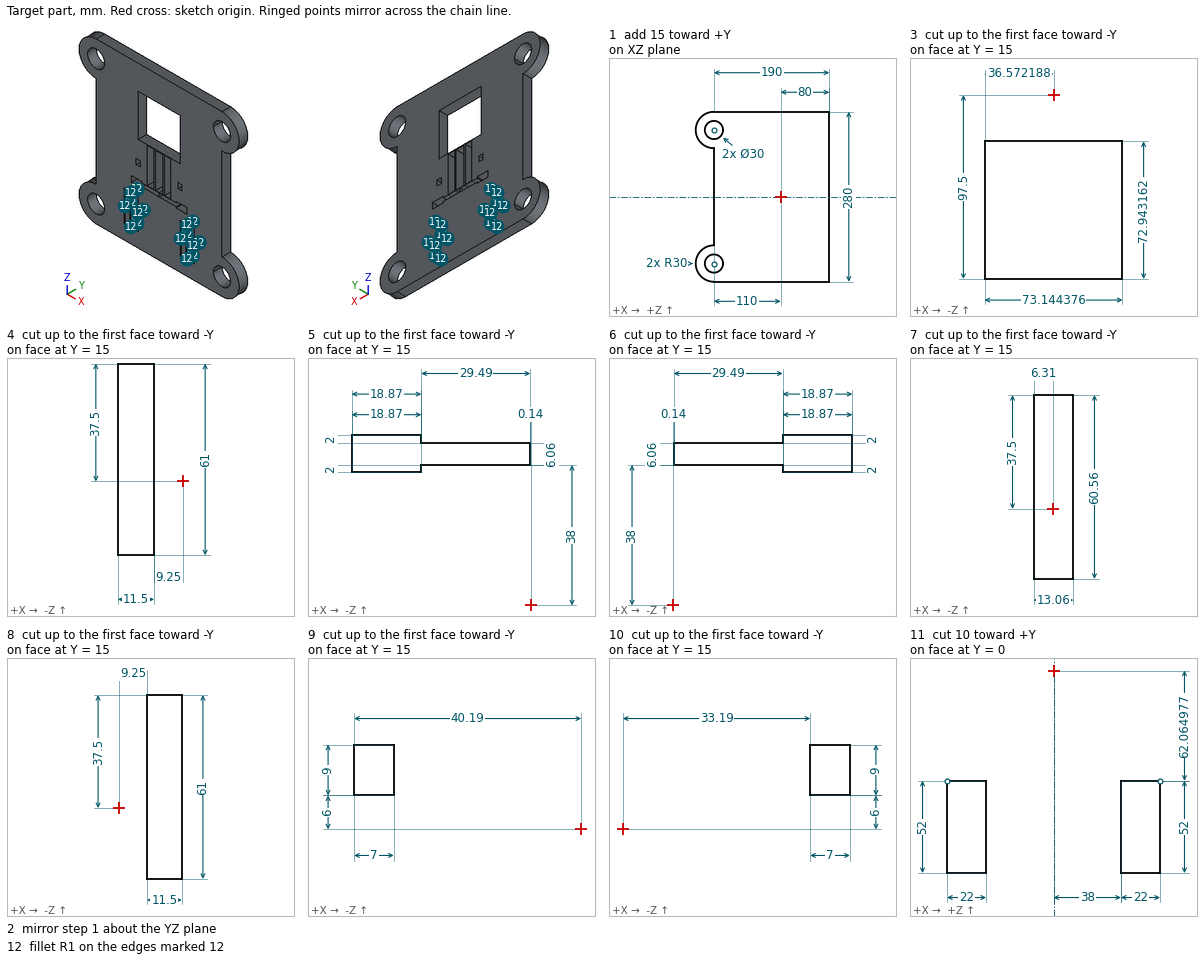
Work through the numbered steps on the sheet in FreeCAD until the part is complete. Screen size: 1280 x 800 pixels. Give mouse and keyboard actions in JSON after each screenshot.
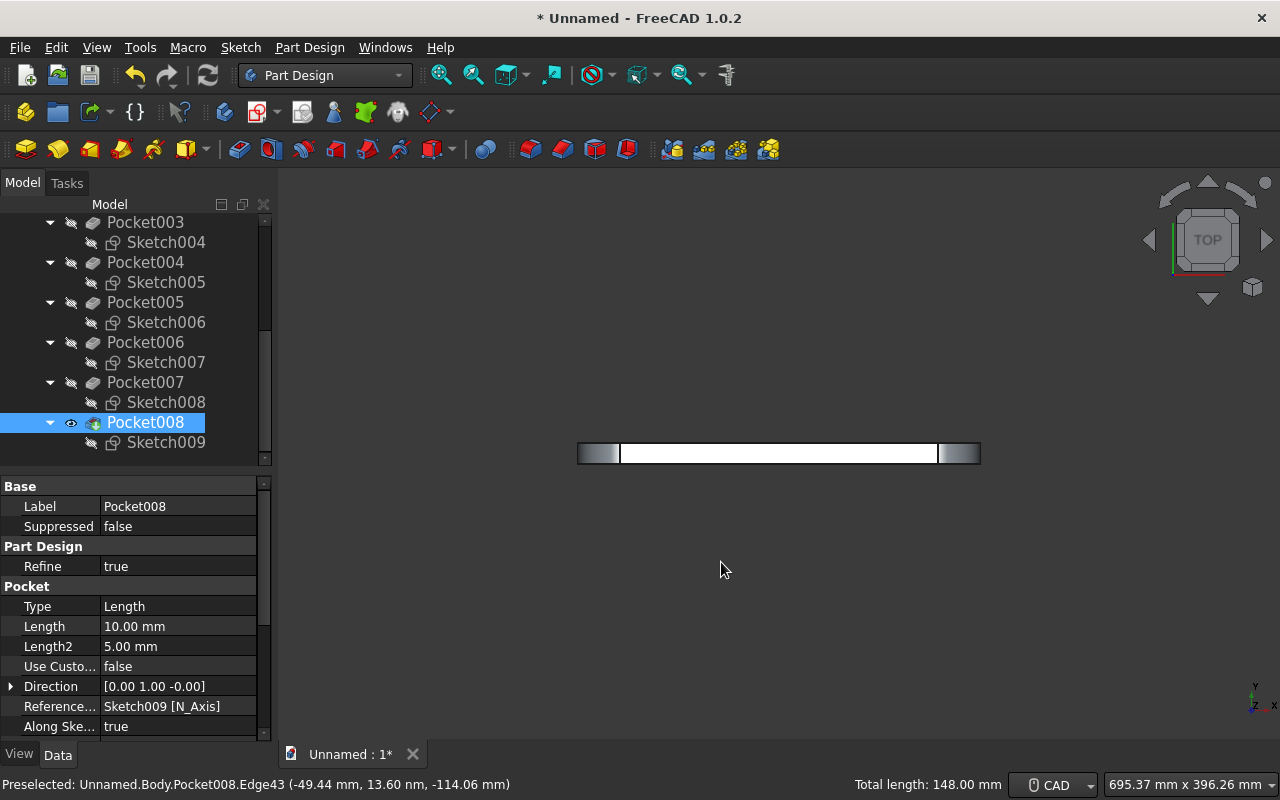
{"action": "left_click", "coordinate": [442, 76]}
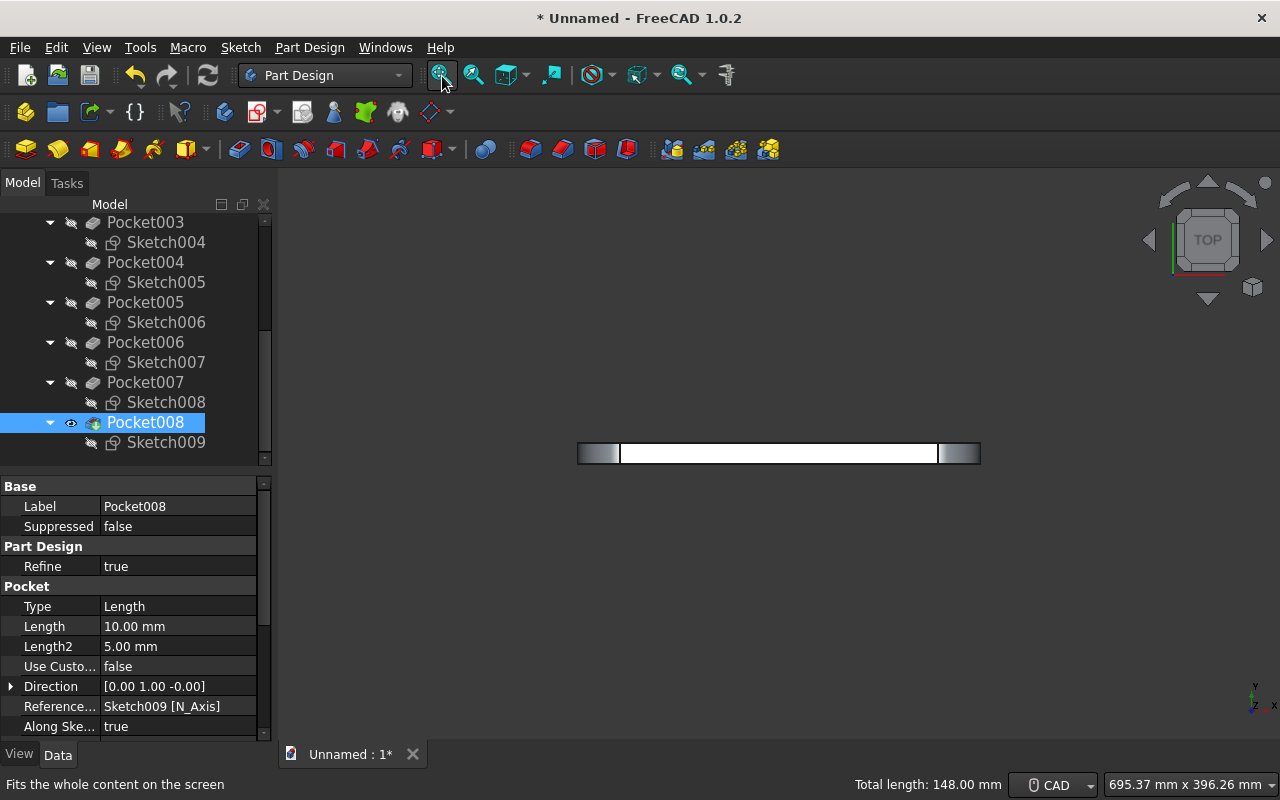
{"action": "key", "text": "0"}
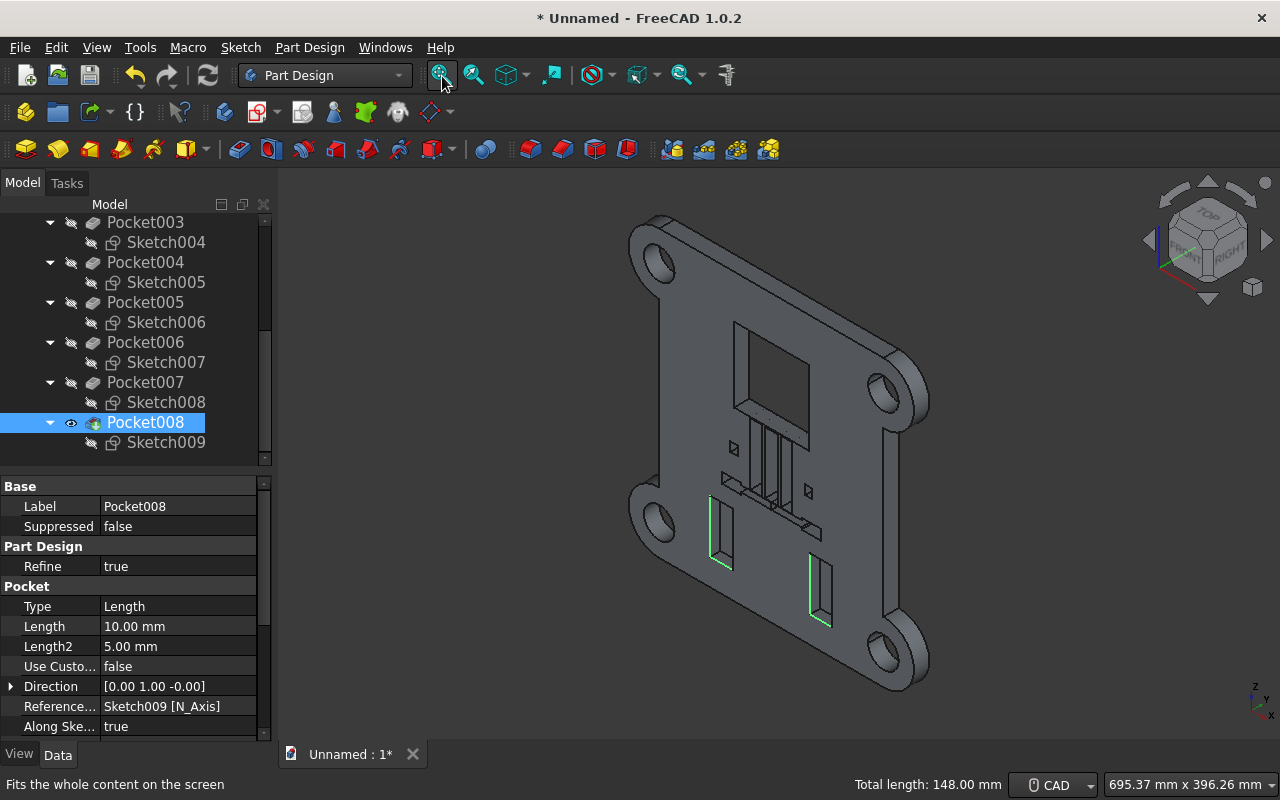
{"action": "key", "text": "1"}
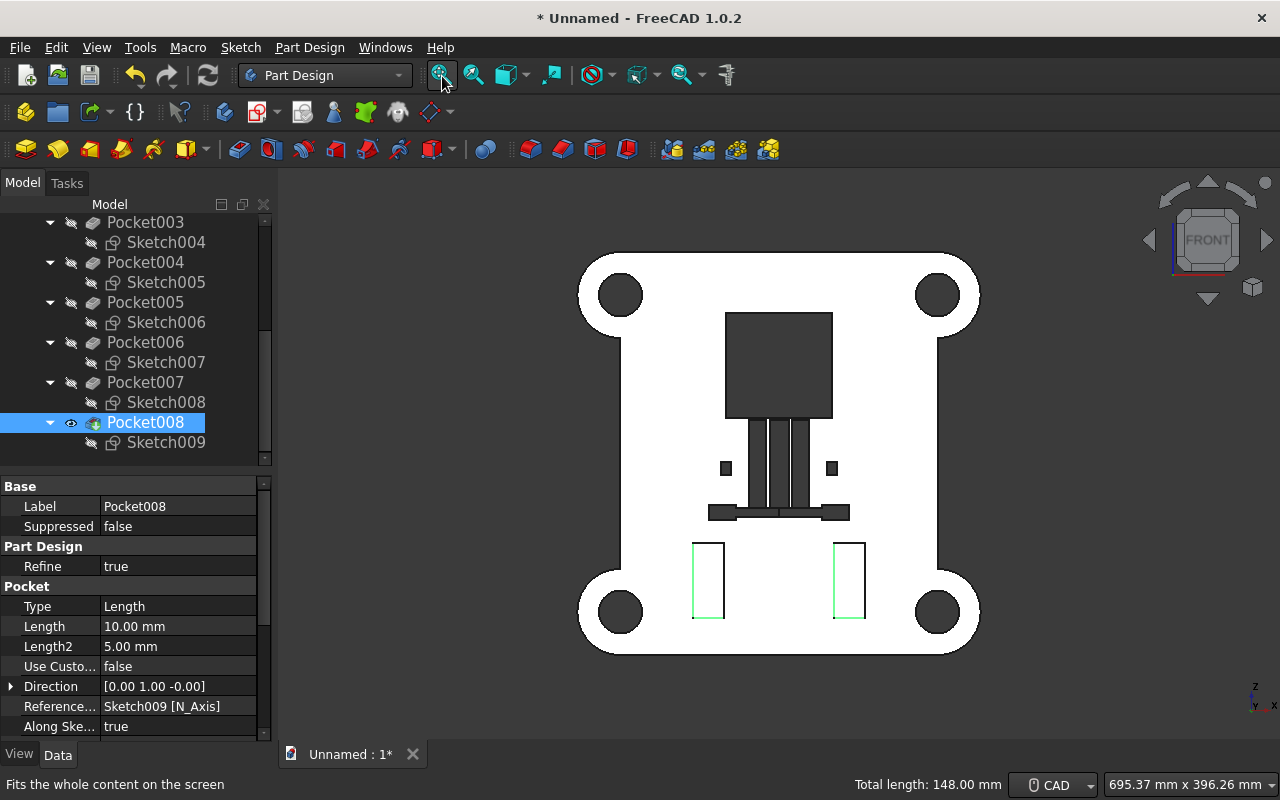
{"action": "left_click", "coordinate": [850, 558], "text": "ctrl"}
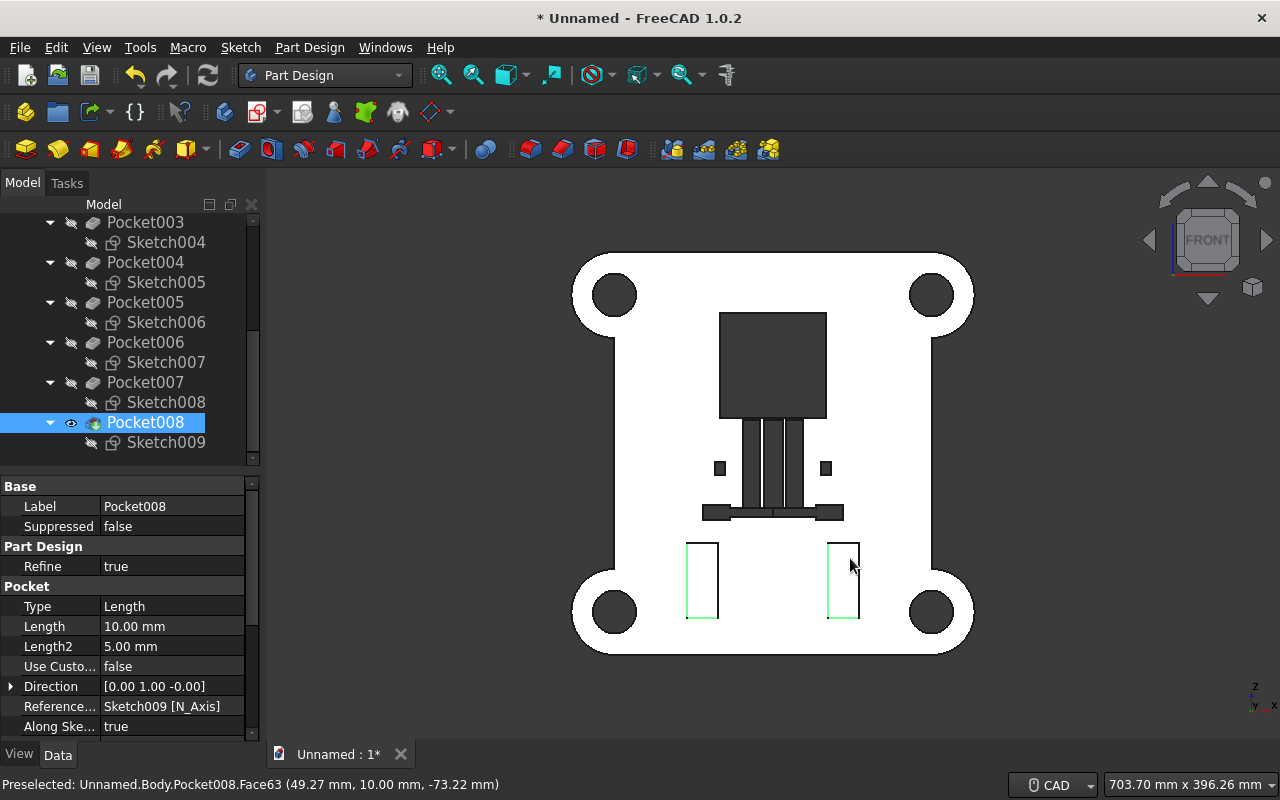
{"action": "left_click", "coordinate": [702, 558], "text": "ctrl"}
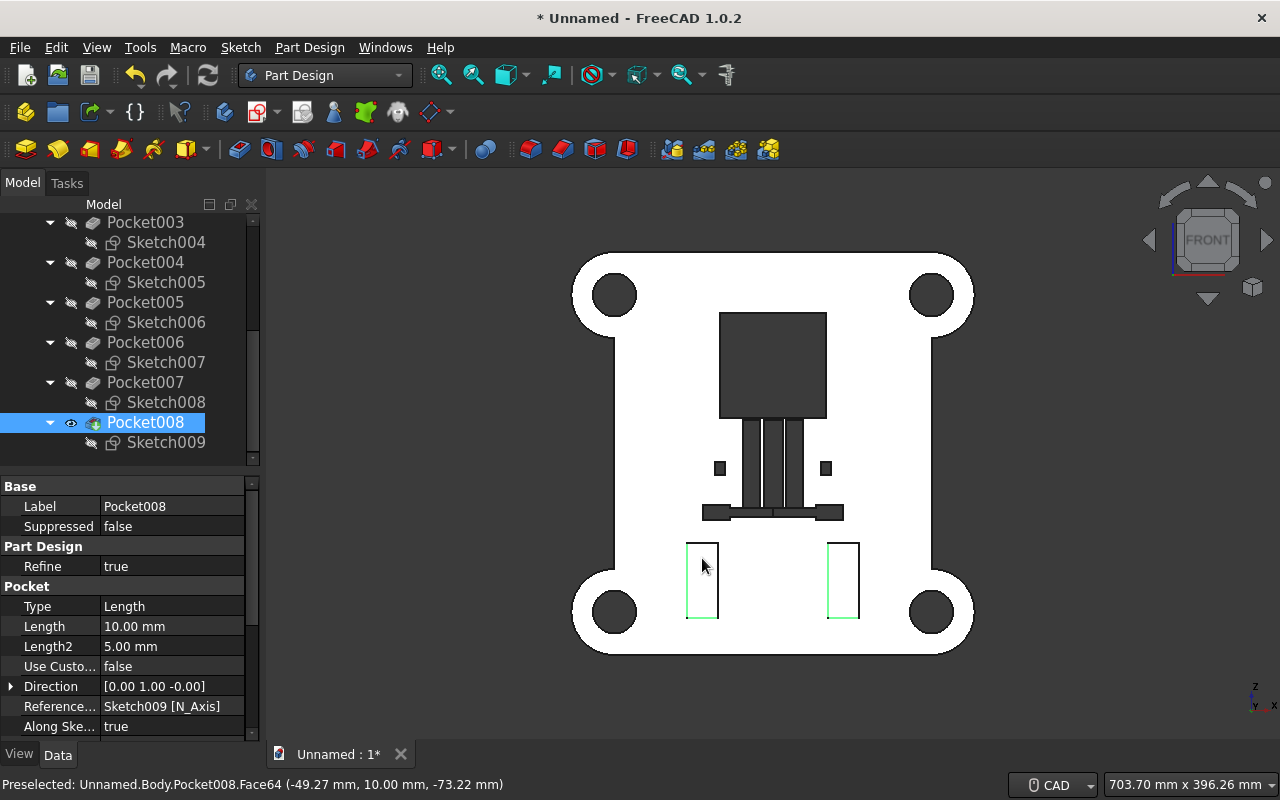
{"action": "left_click", "coordinate": [718, 579], "text": "ctrl"}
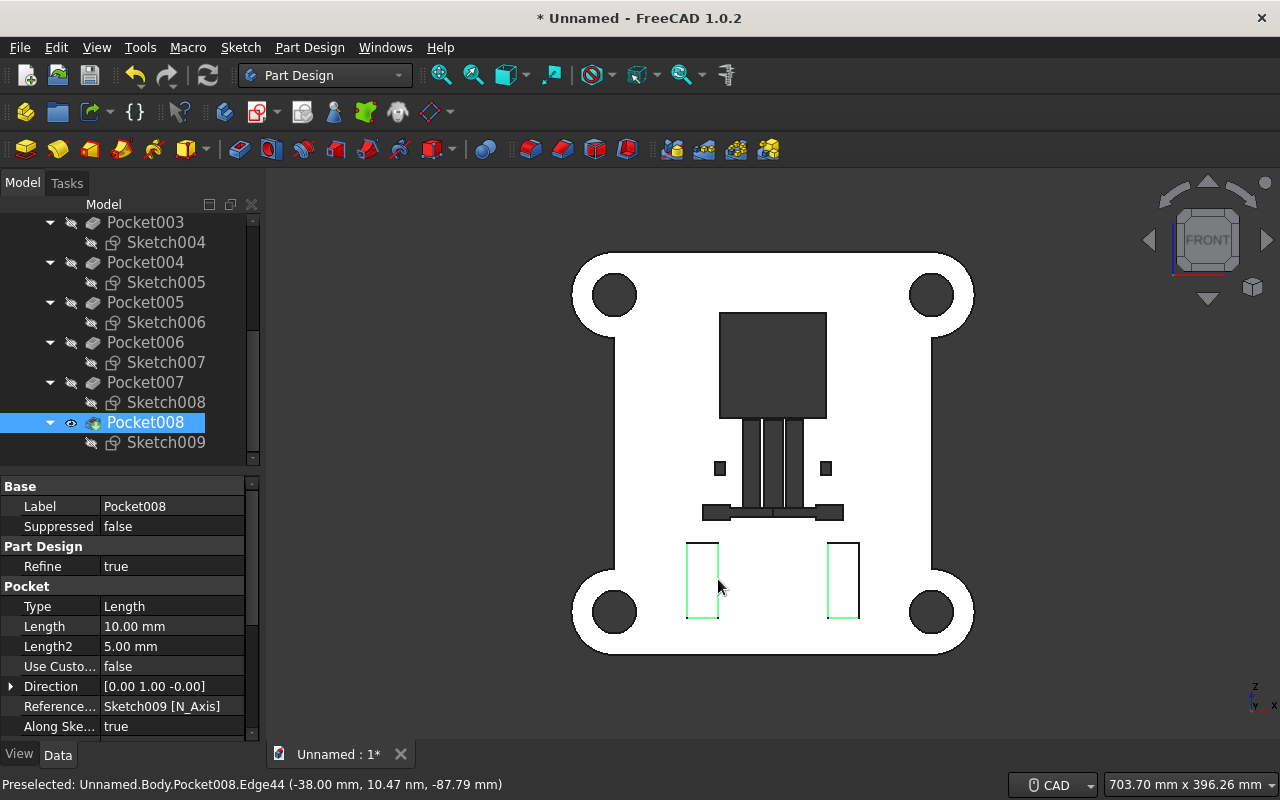
{"action": "key", "text": "3"}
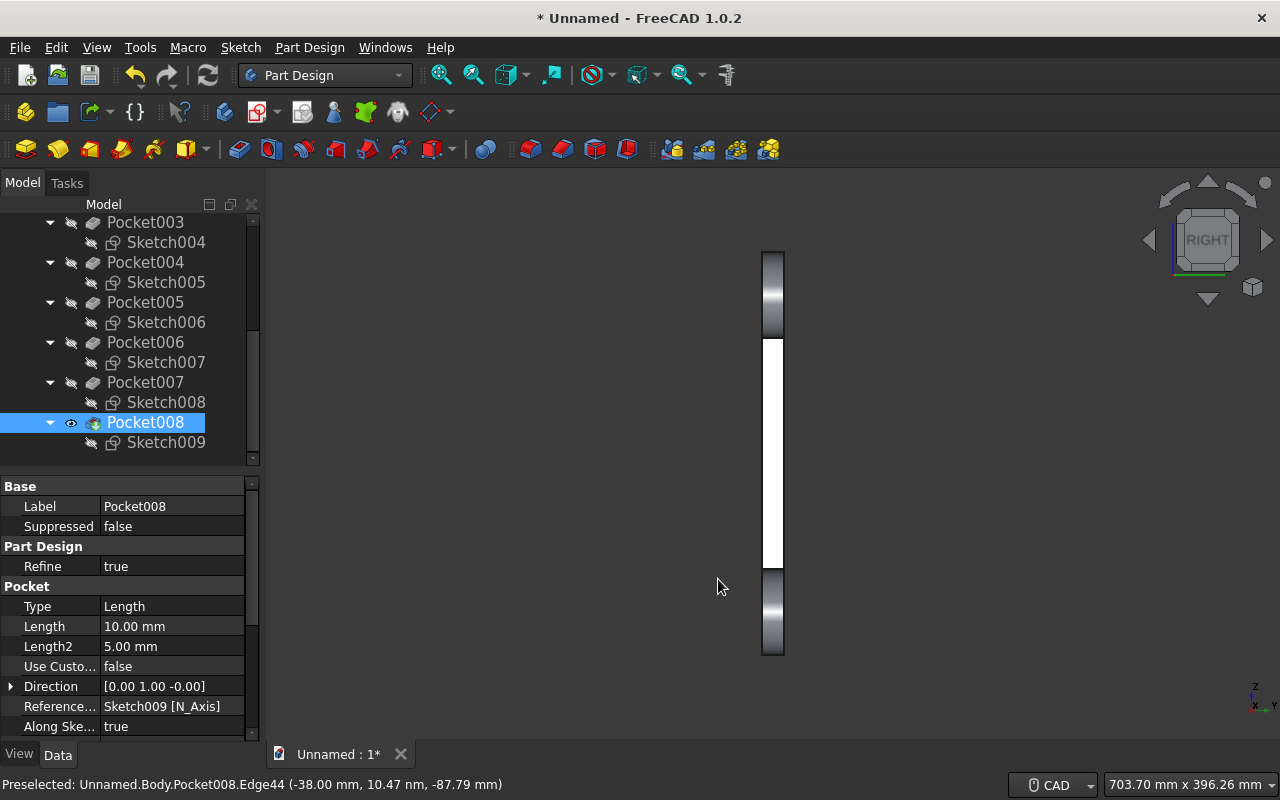
{"action": "key", "text": "5"}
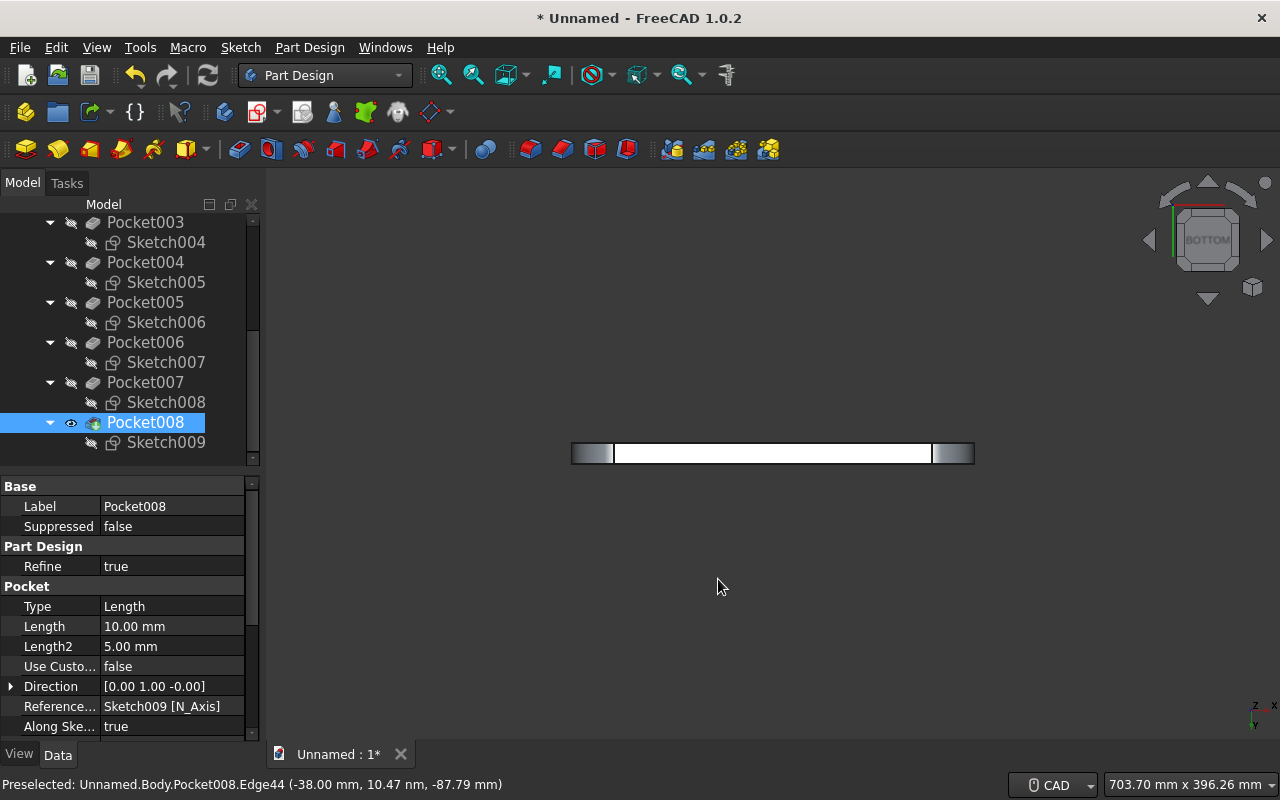
{"action": "left_click", "coordinate": [442, 76]}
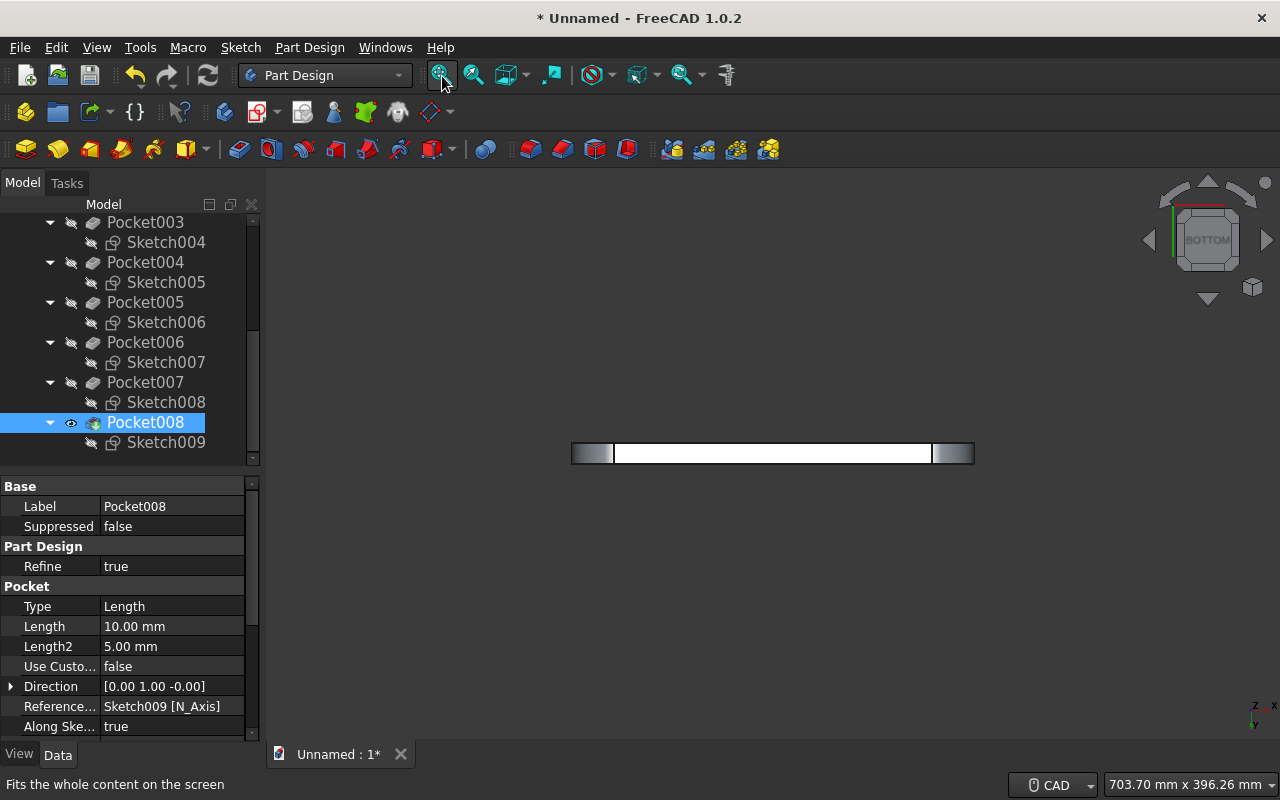
{"action": "key", "text": "4"}